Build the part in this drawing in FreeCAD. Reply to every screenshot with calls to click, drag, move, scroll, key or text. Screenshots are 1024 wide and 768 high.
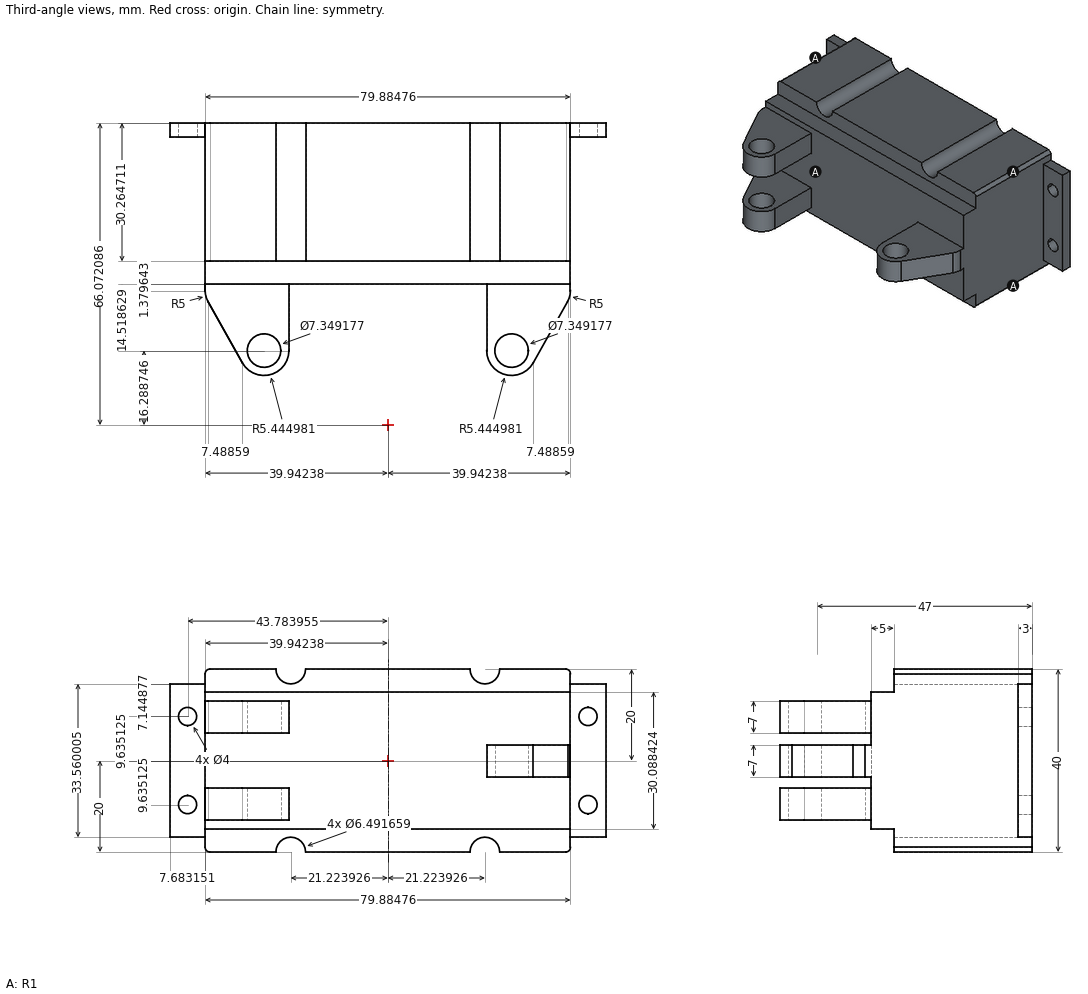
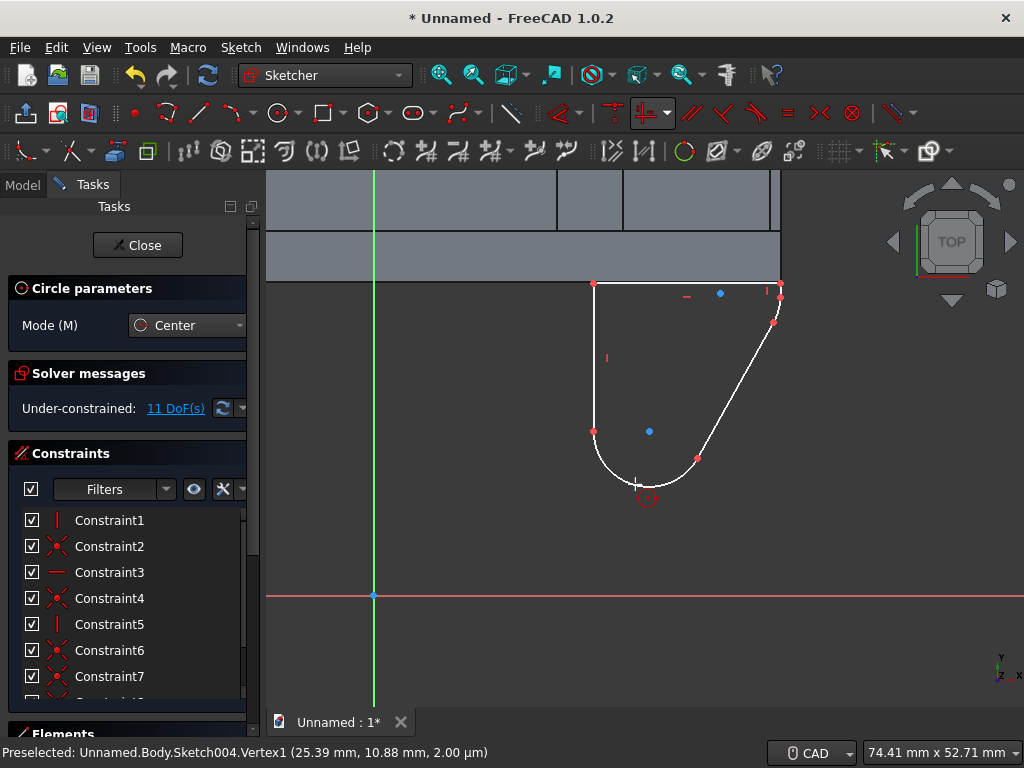
click(649, 430)
click(676, 403)
key(Escape)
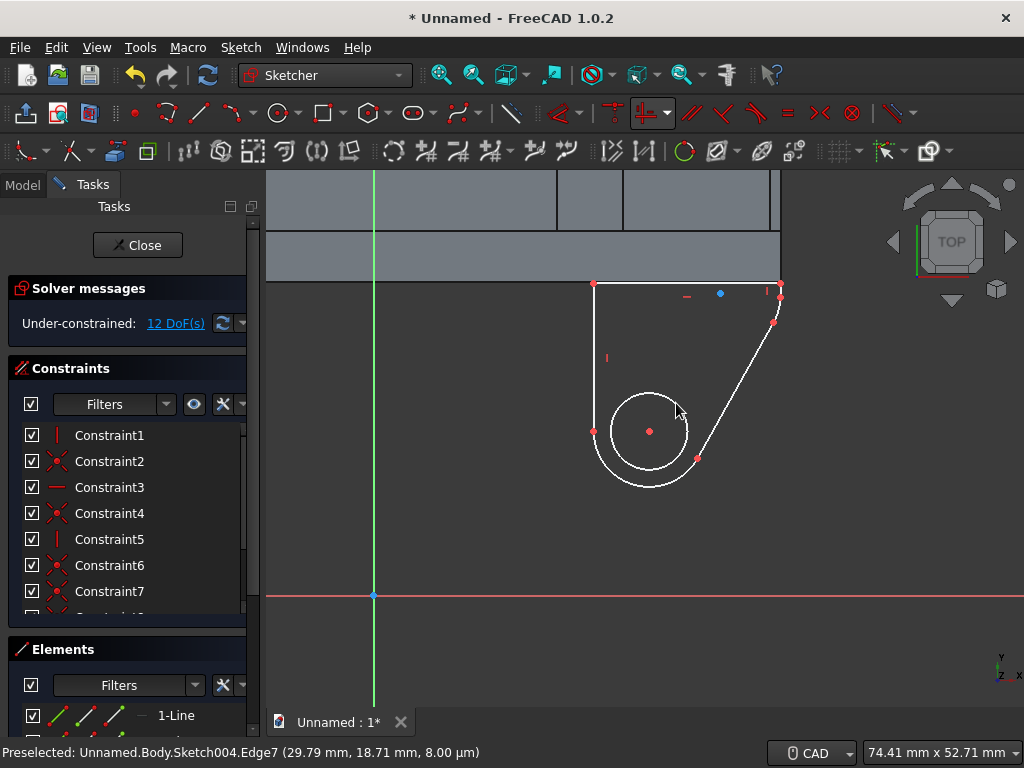
click(721, 417)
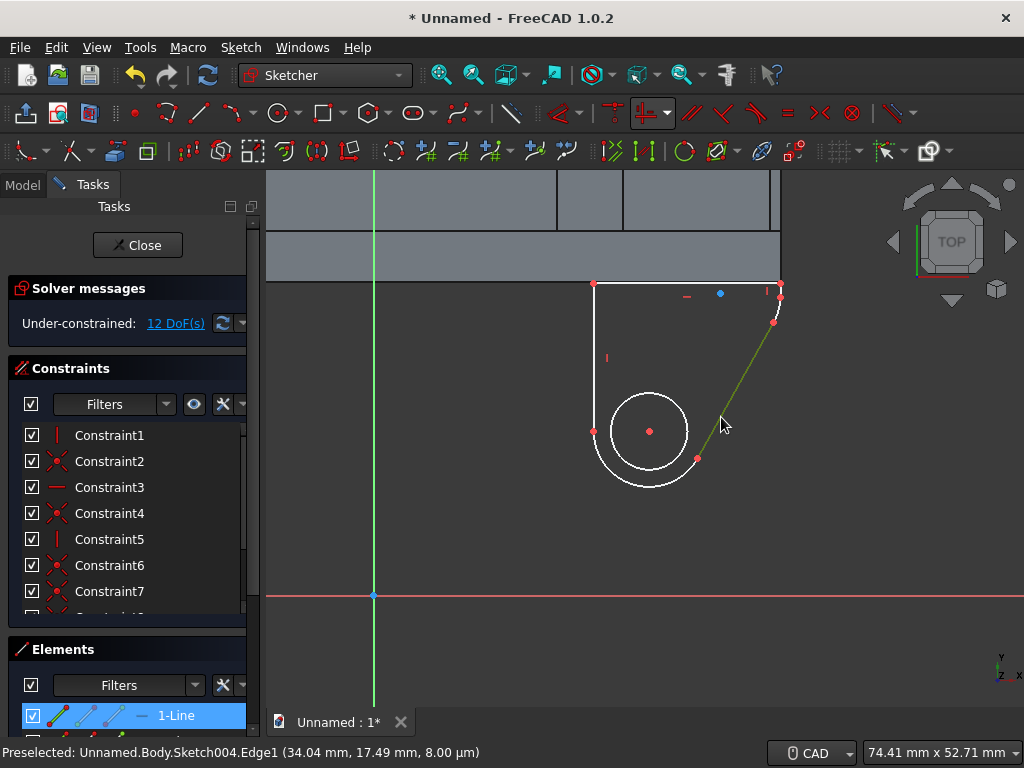
click(779, 310)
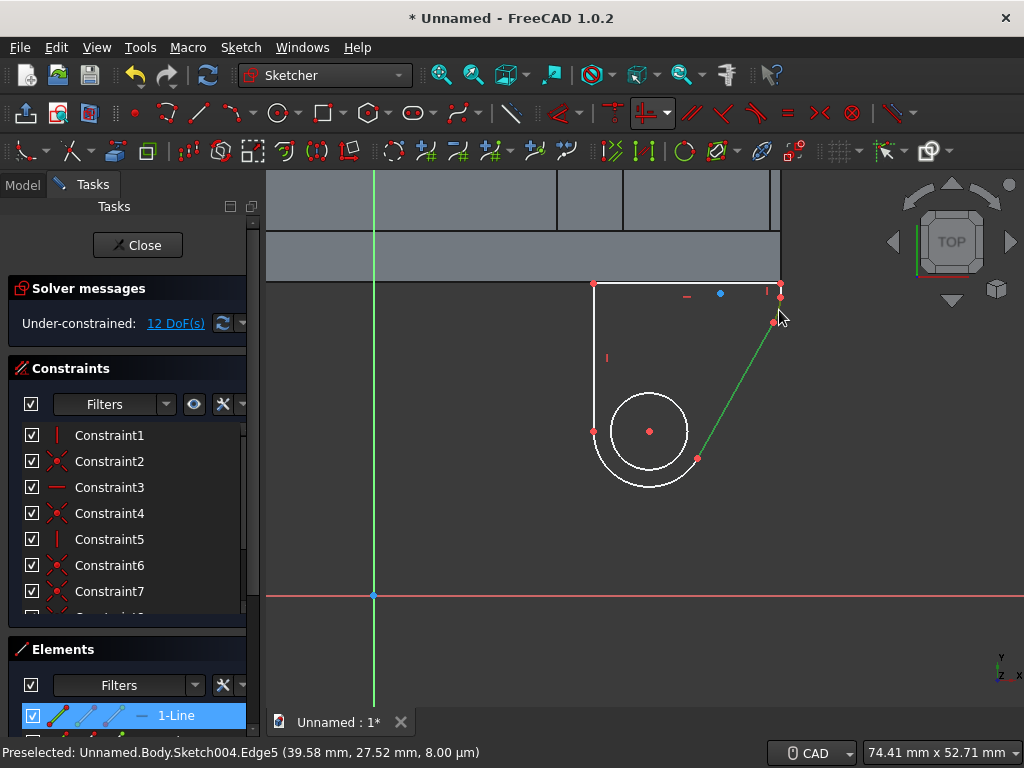
click(756, 114)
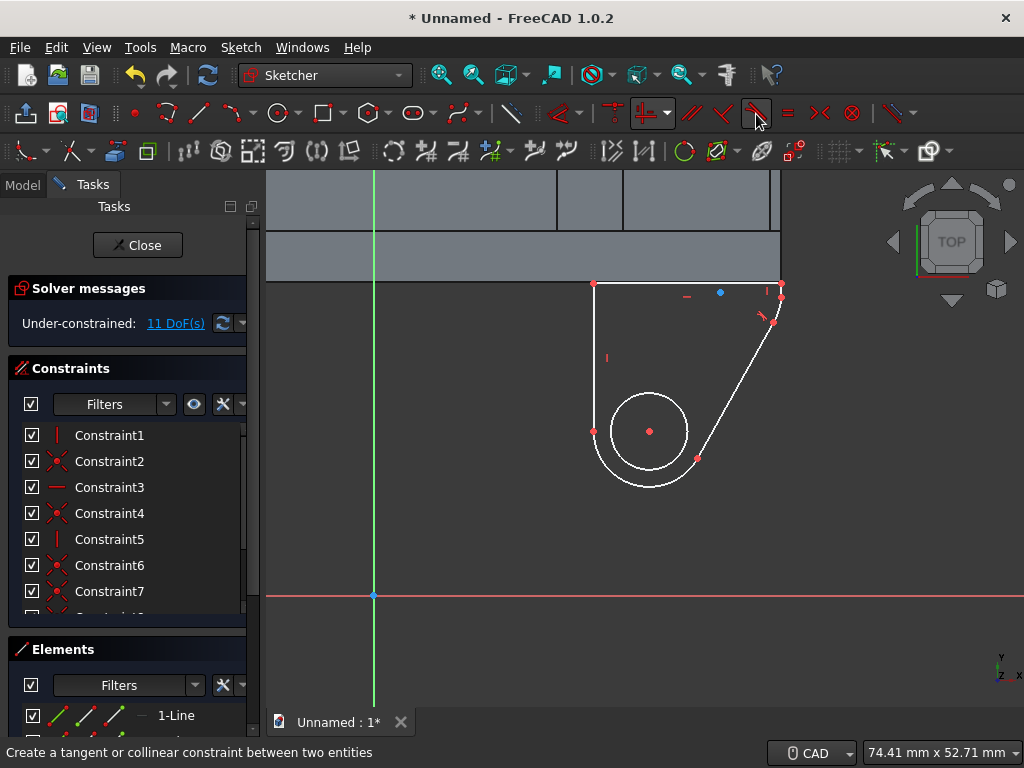
click(721, 417)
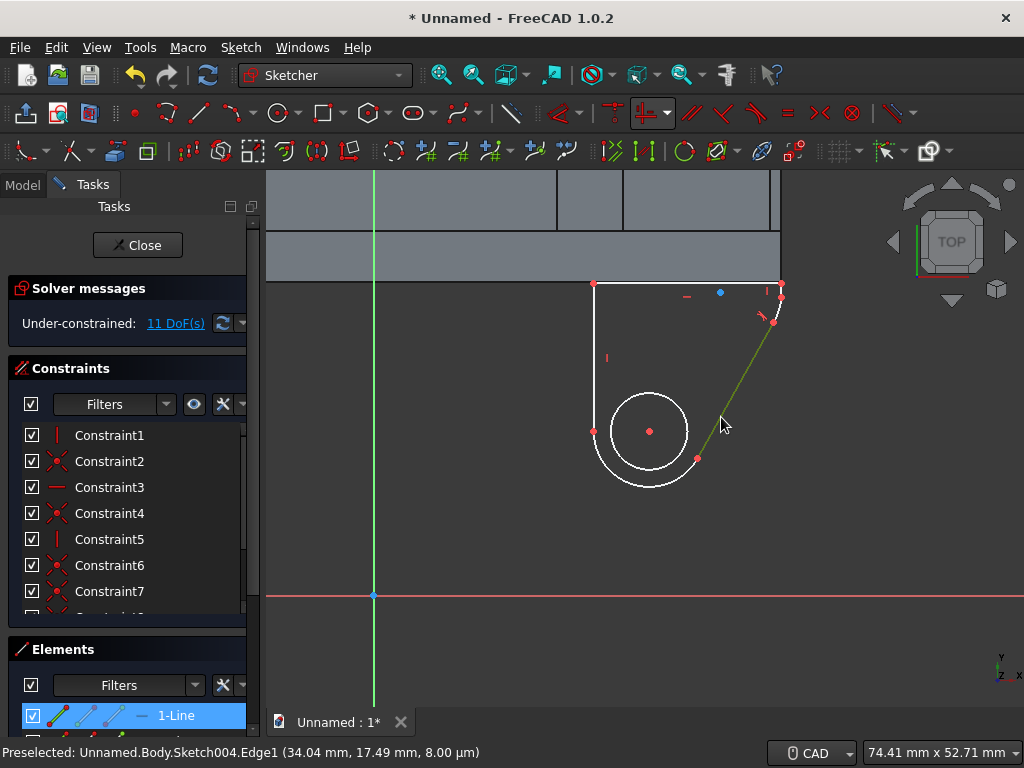
click(610, 471)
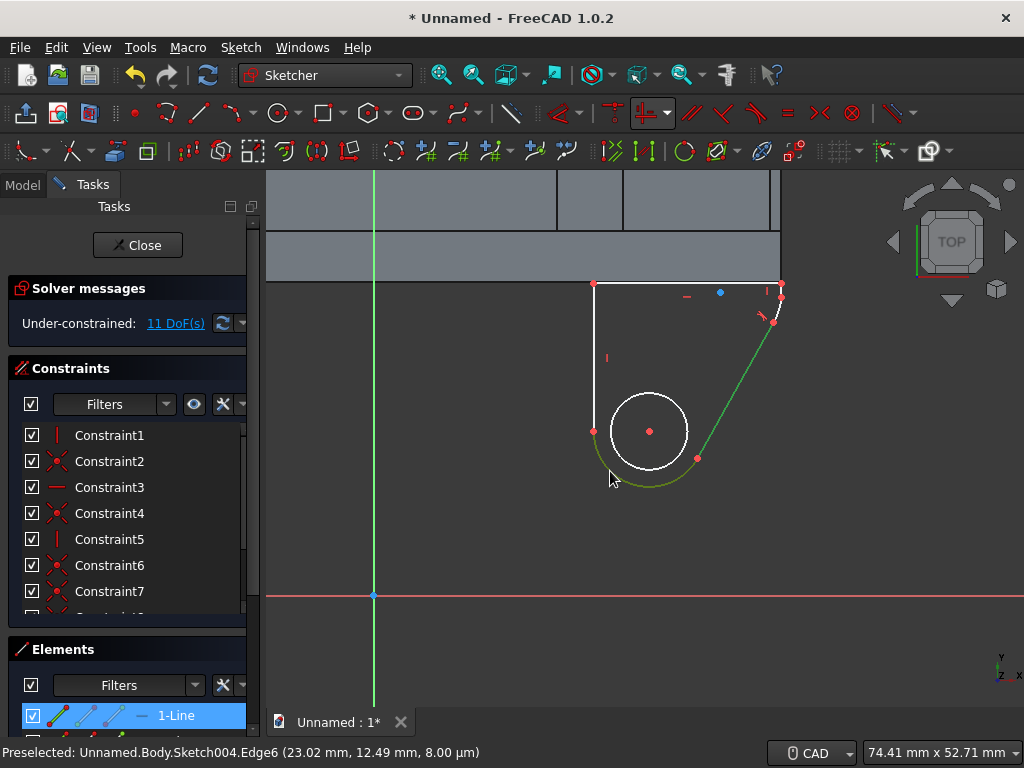
click(756, 114)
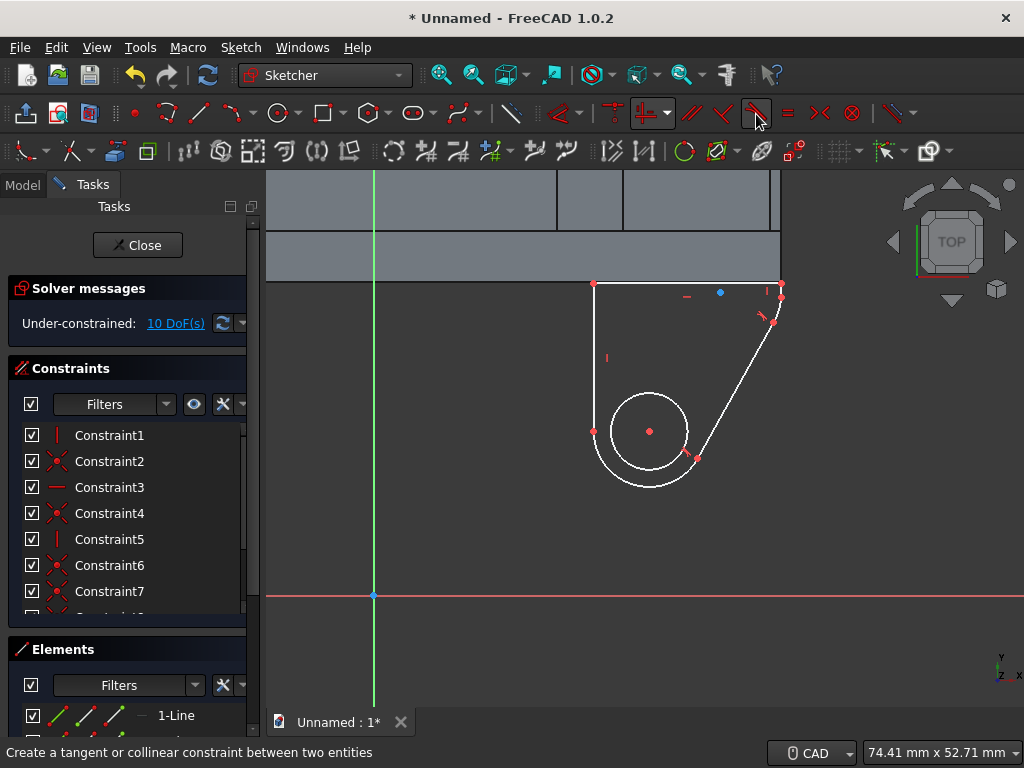
scroll(781, 290, up, 4)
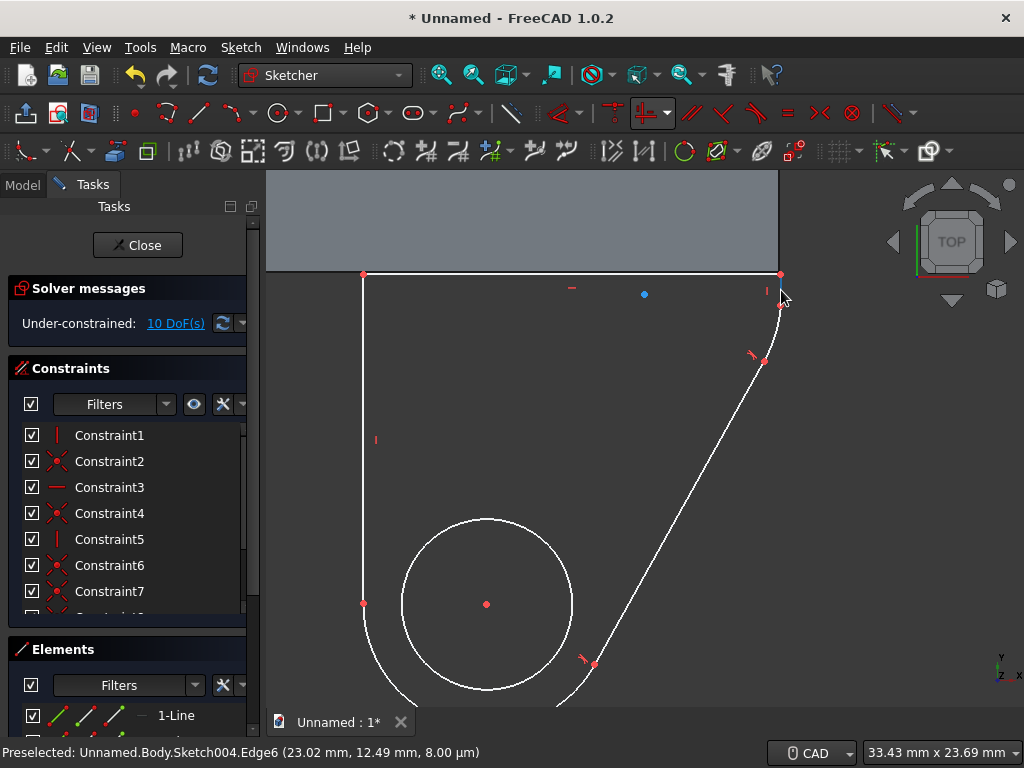
click(781, 290)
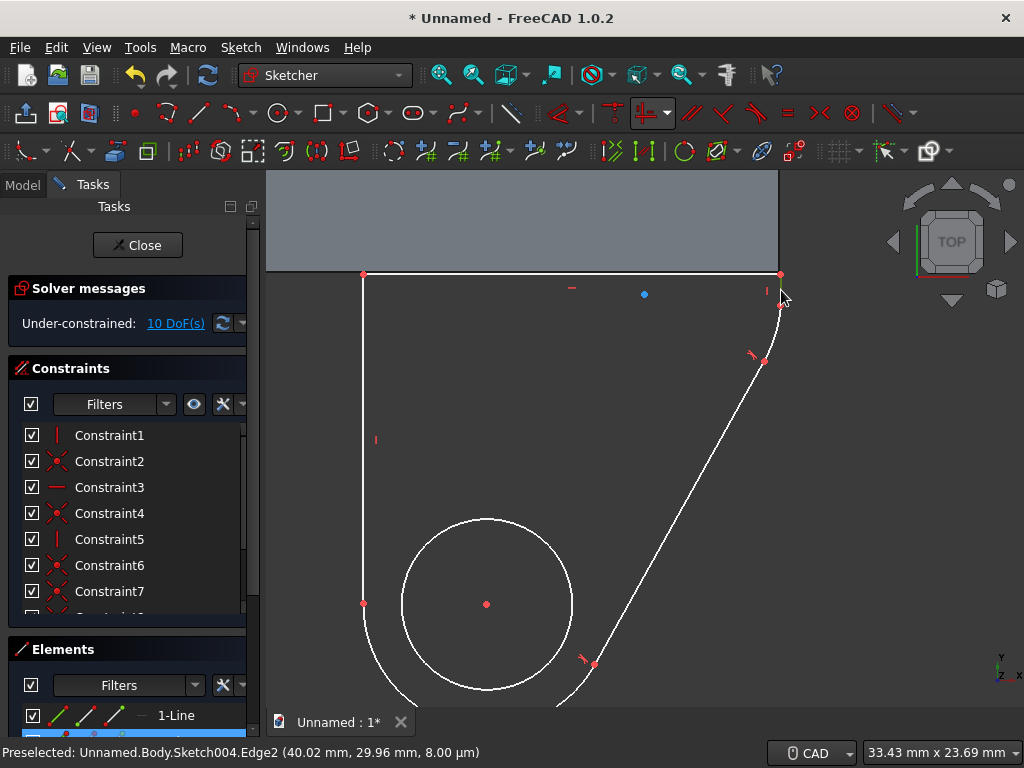
click(772, 345)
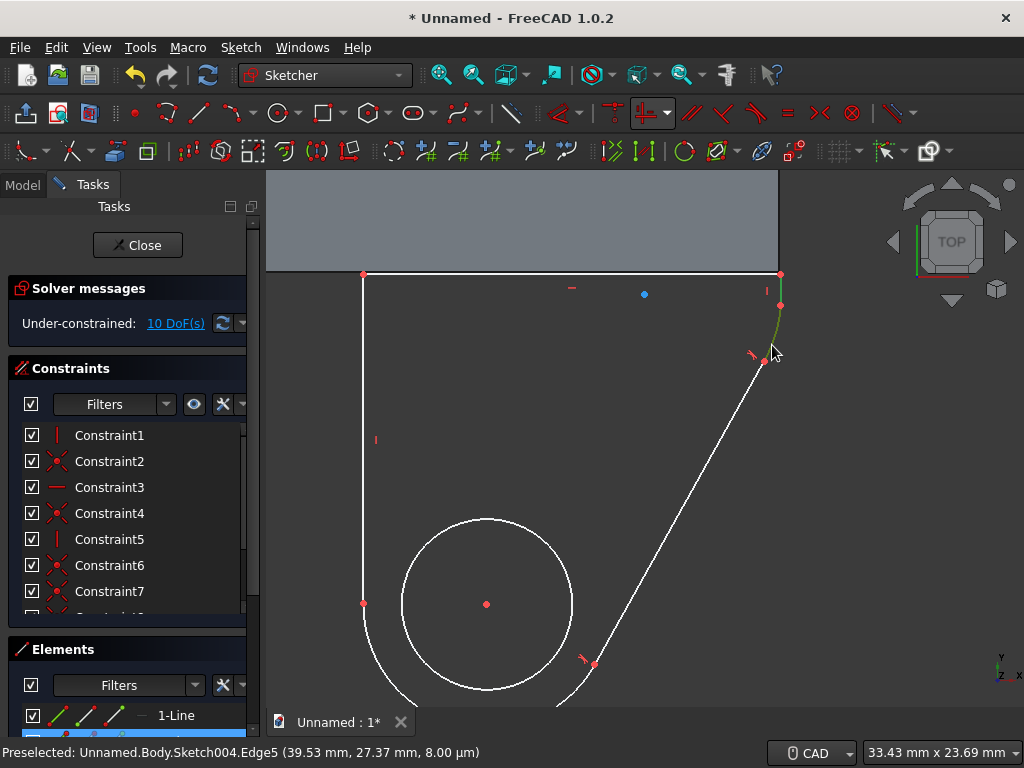
click(756, 114)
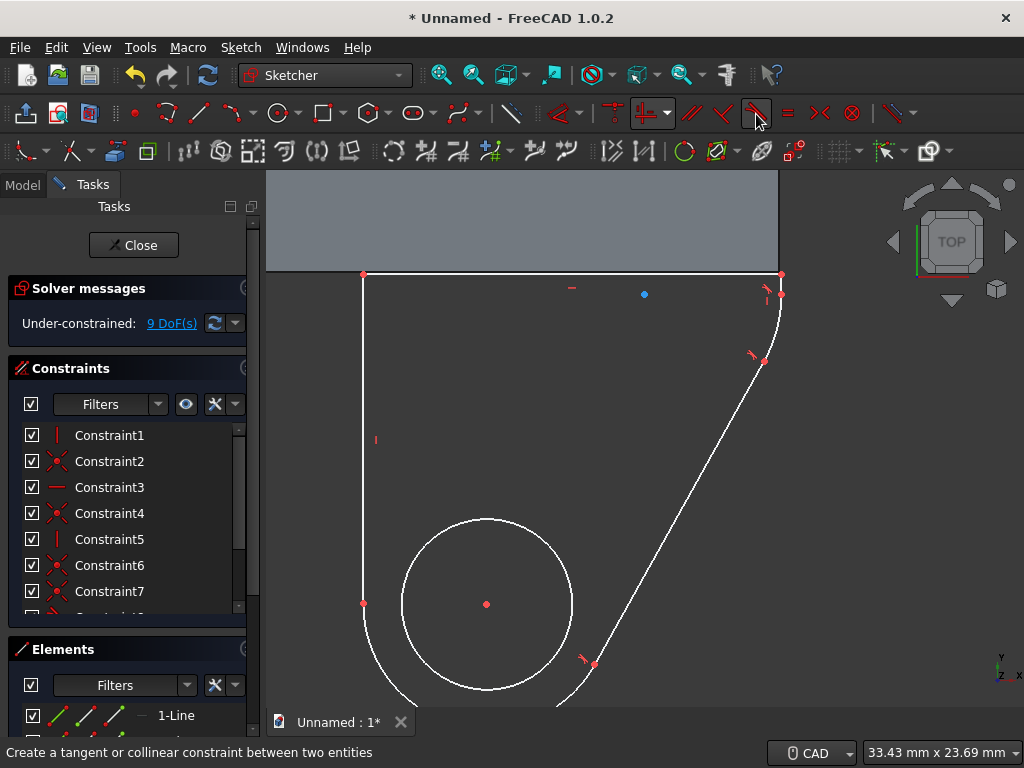
click(363, 373)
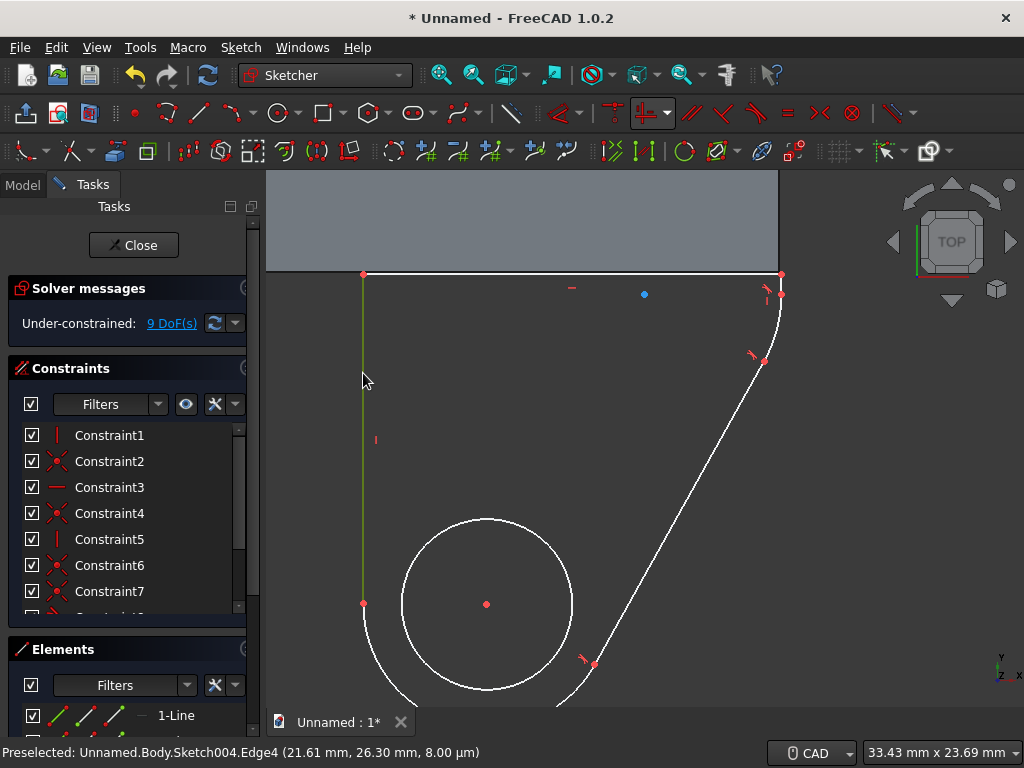
click(380, 666)